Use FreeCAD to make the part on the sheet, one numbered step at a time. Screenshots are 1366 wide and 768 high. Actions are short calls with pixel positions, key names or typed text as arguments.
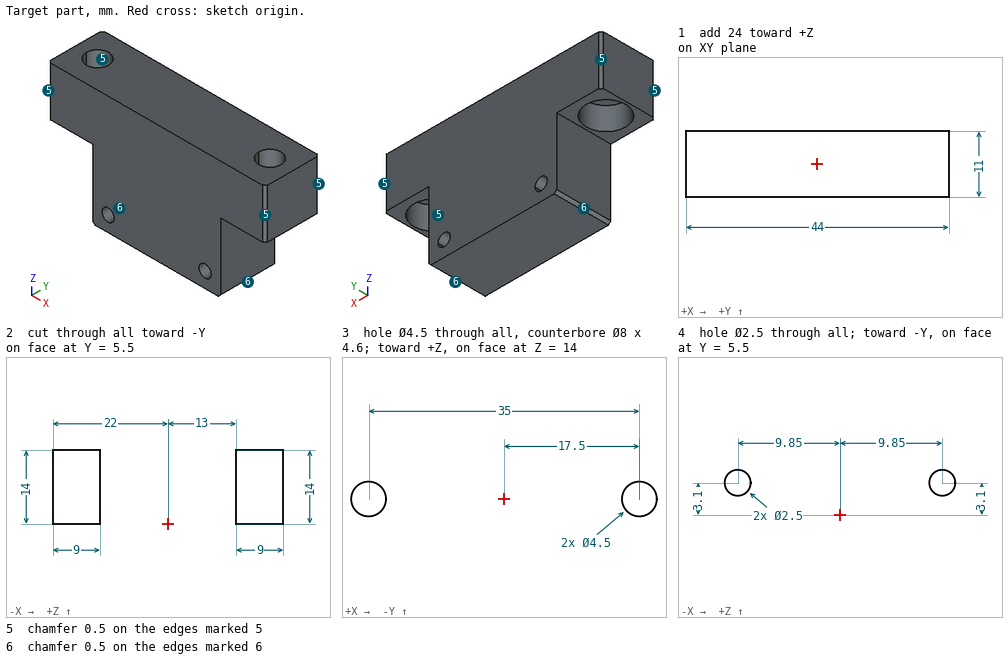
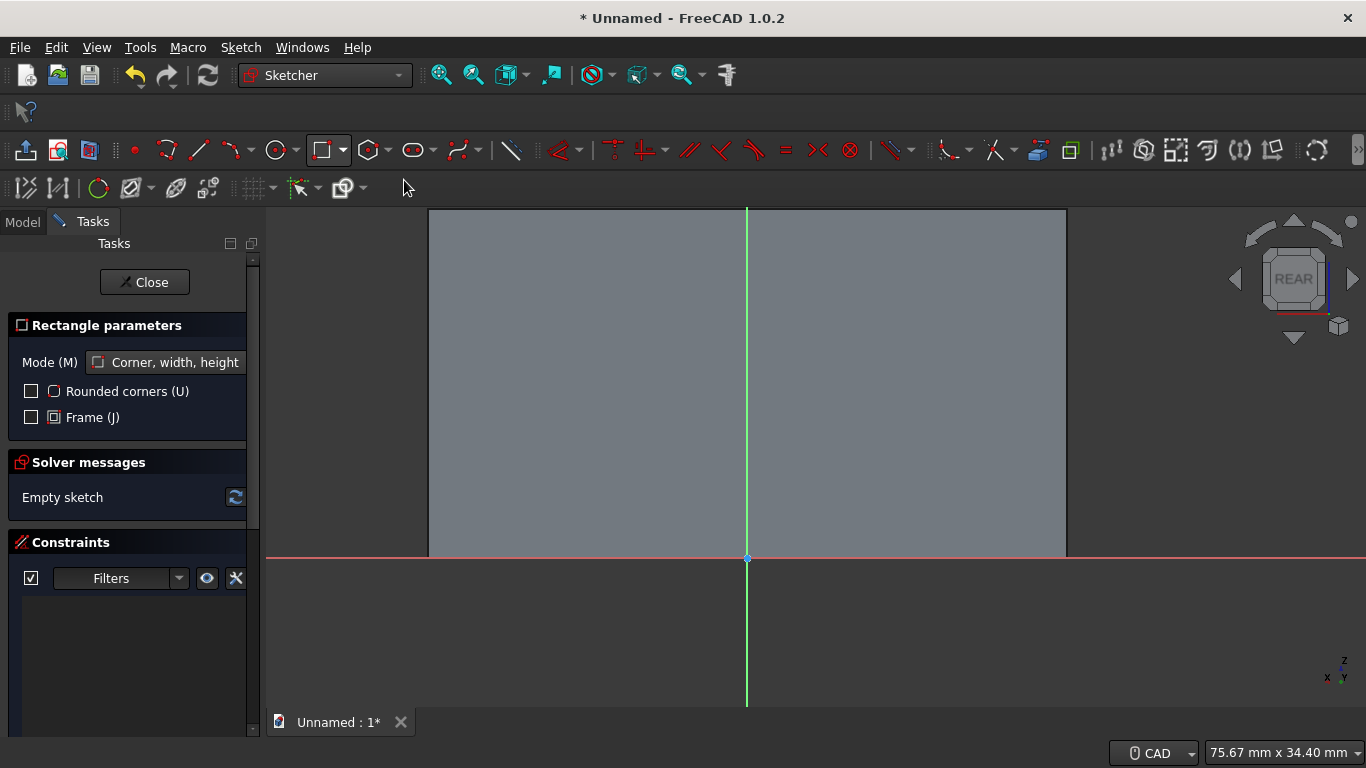
click(936, 355)
click(1067, 558)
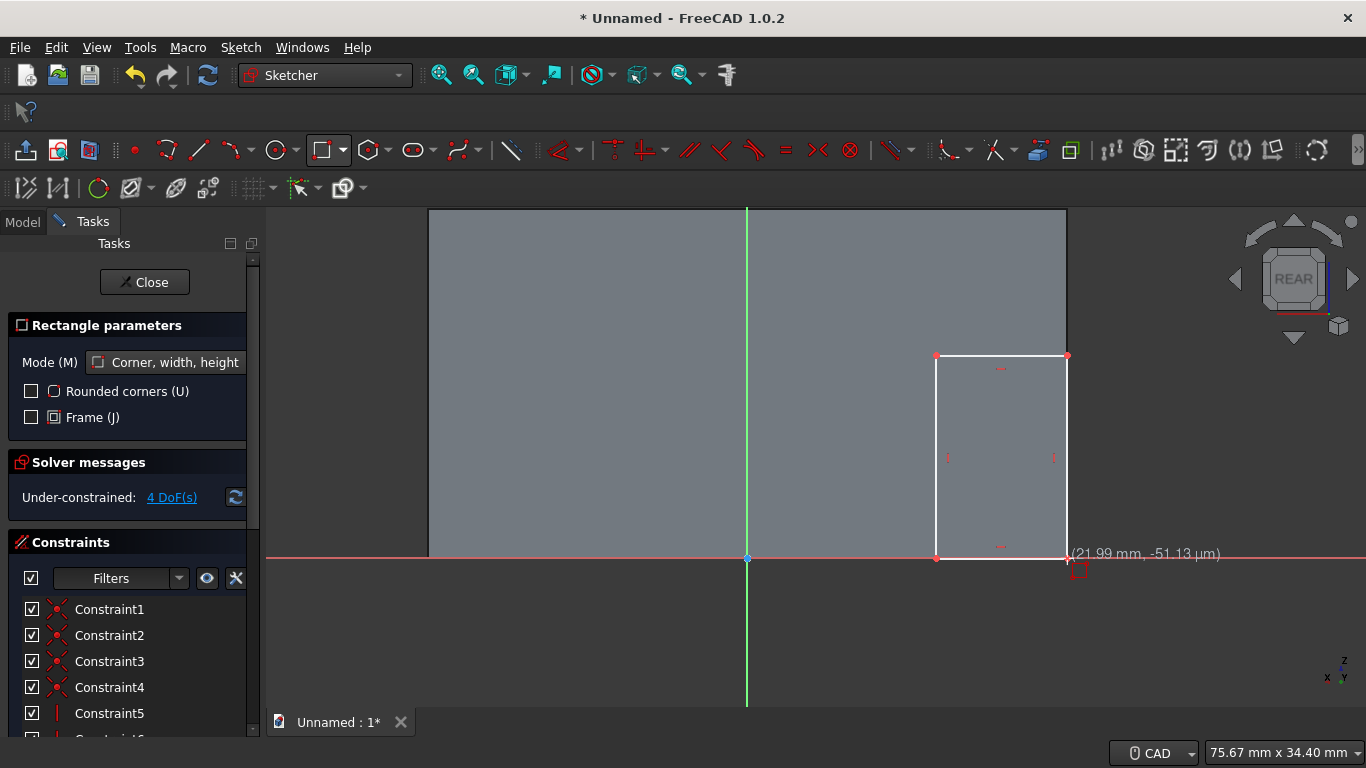
click(428, 355)
click(558, 558)
key(Escape)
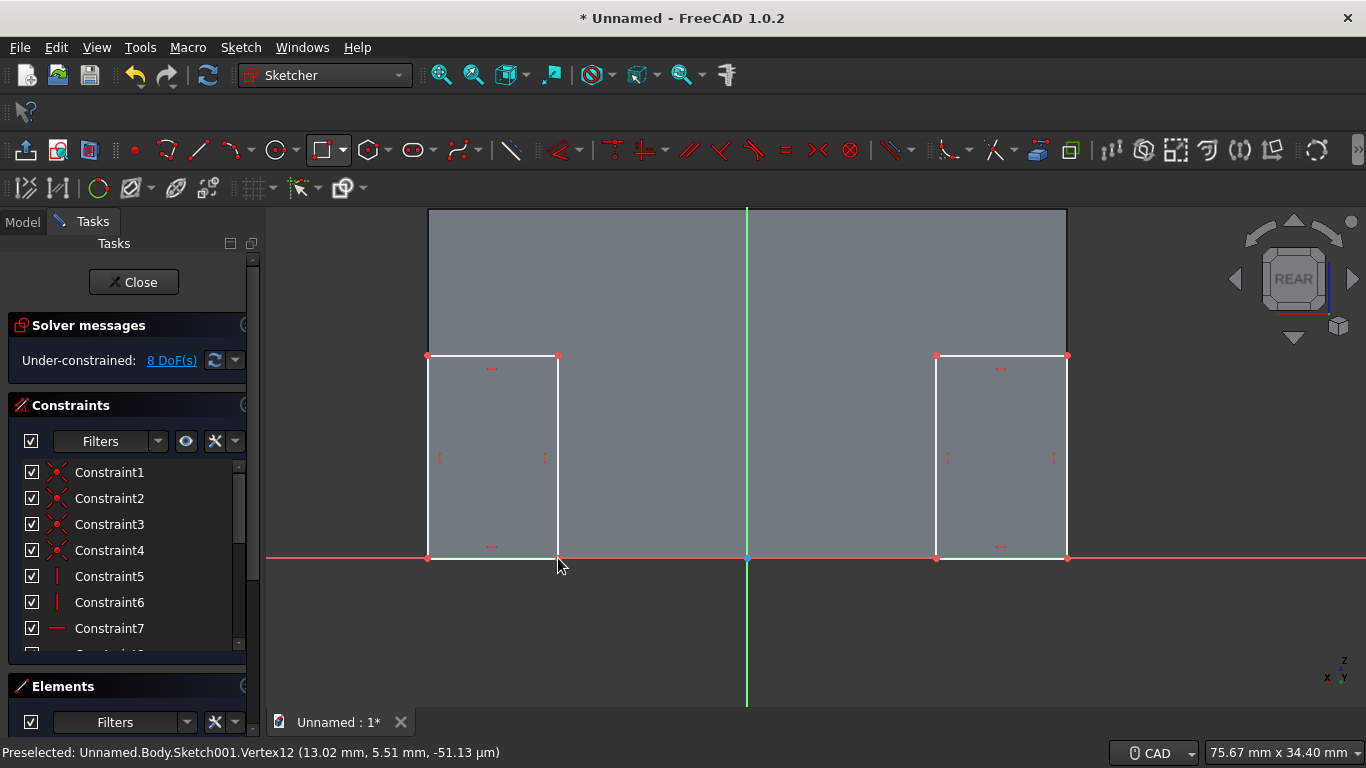
click(936, 559)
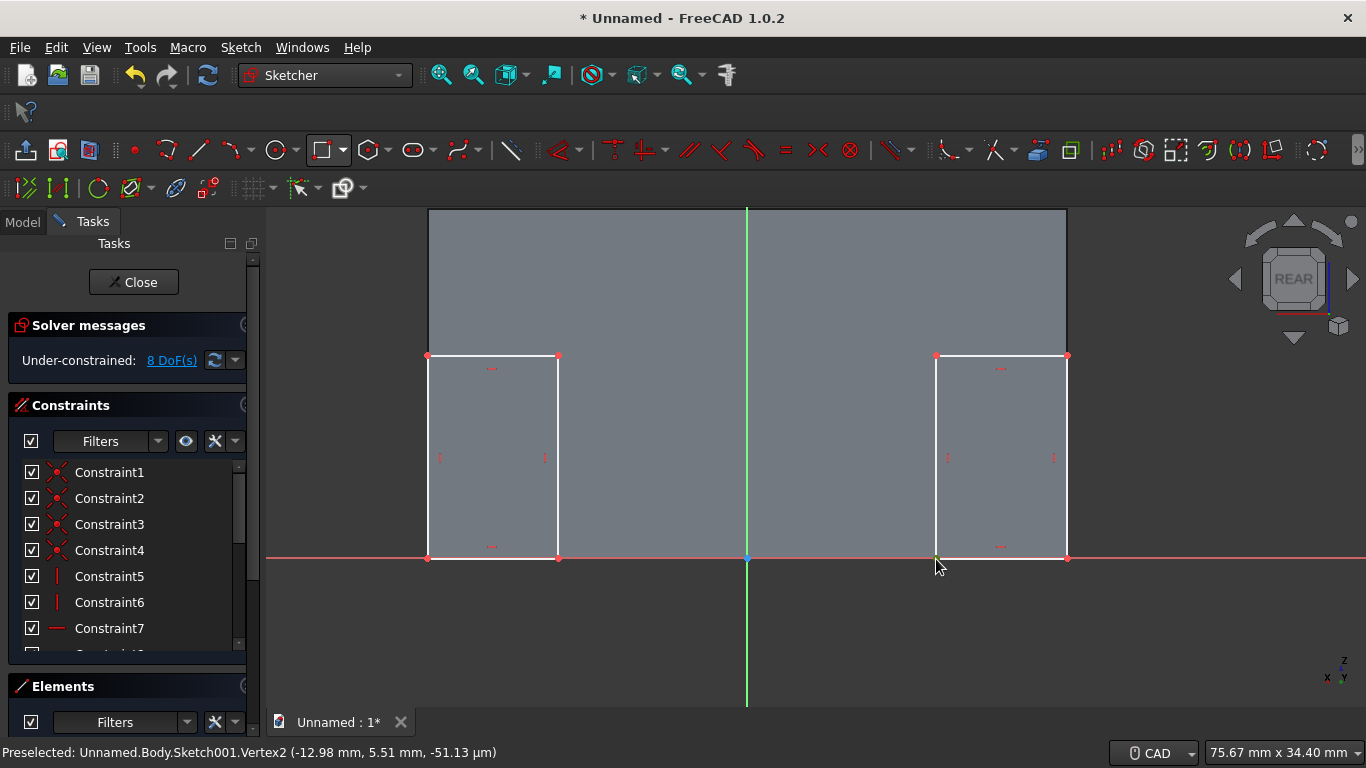
click(359, 558)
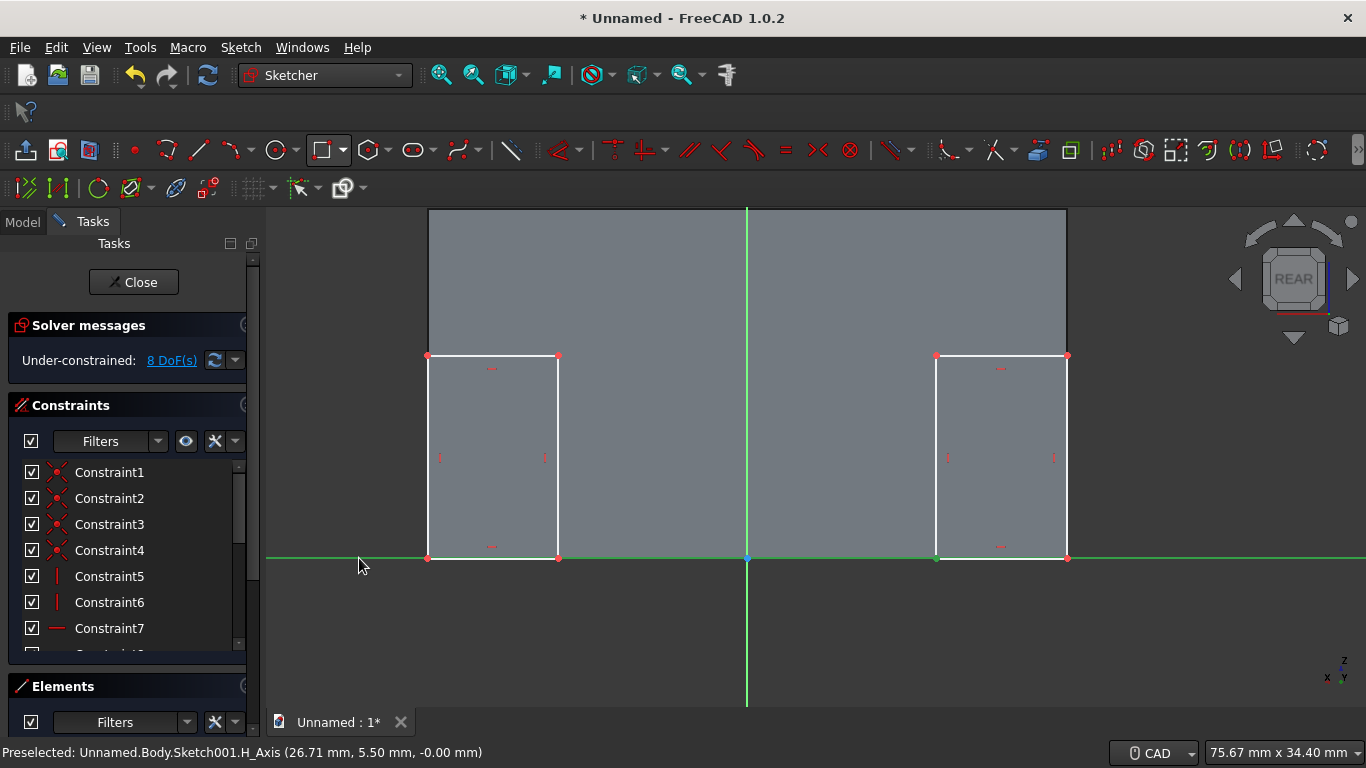
click(614, 150)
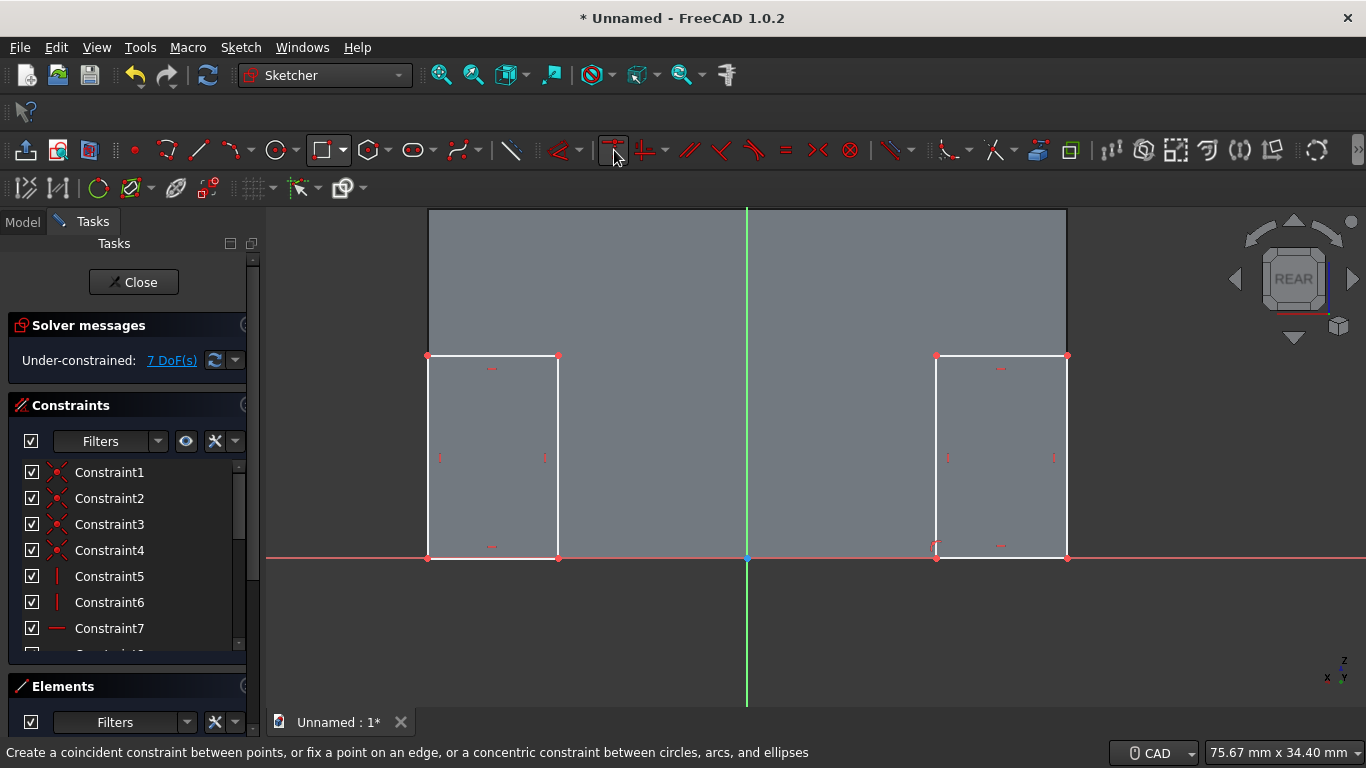
click(428, 559)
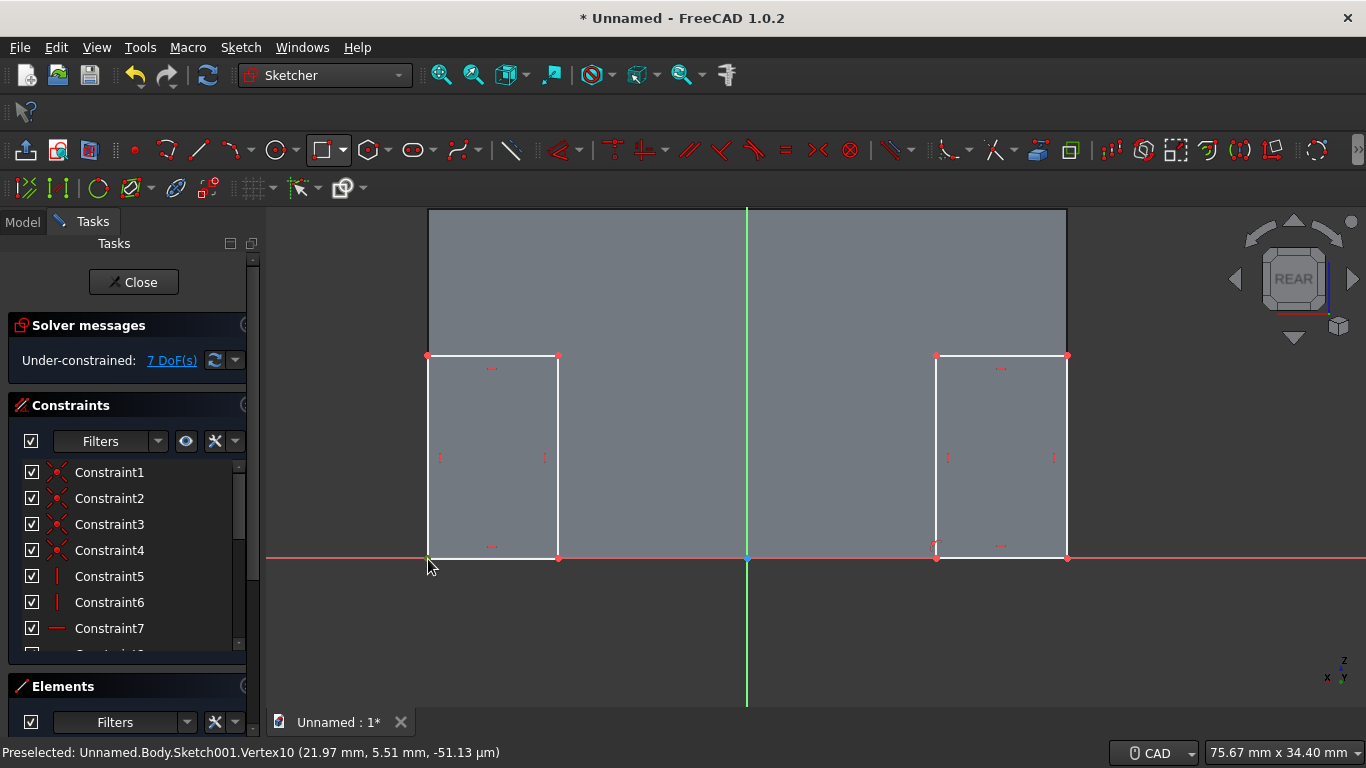
click(359, 558)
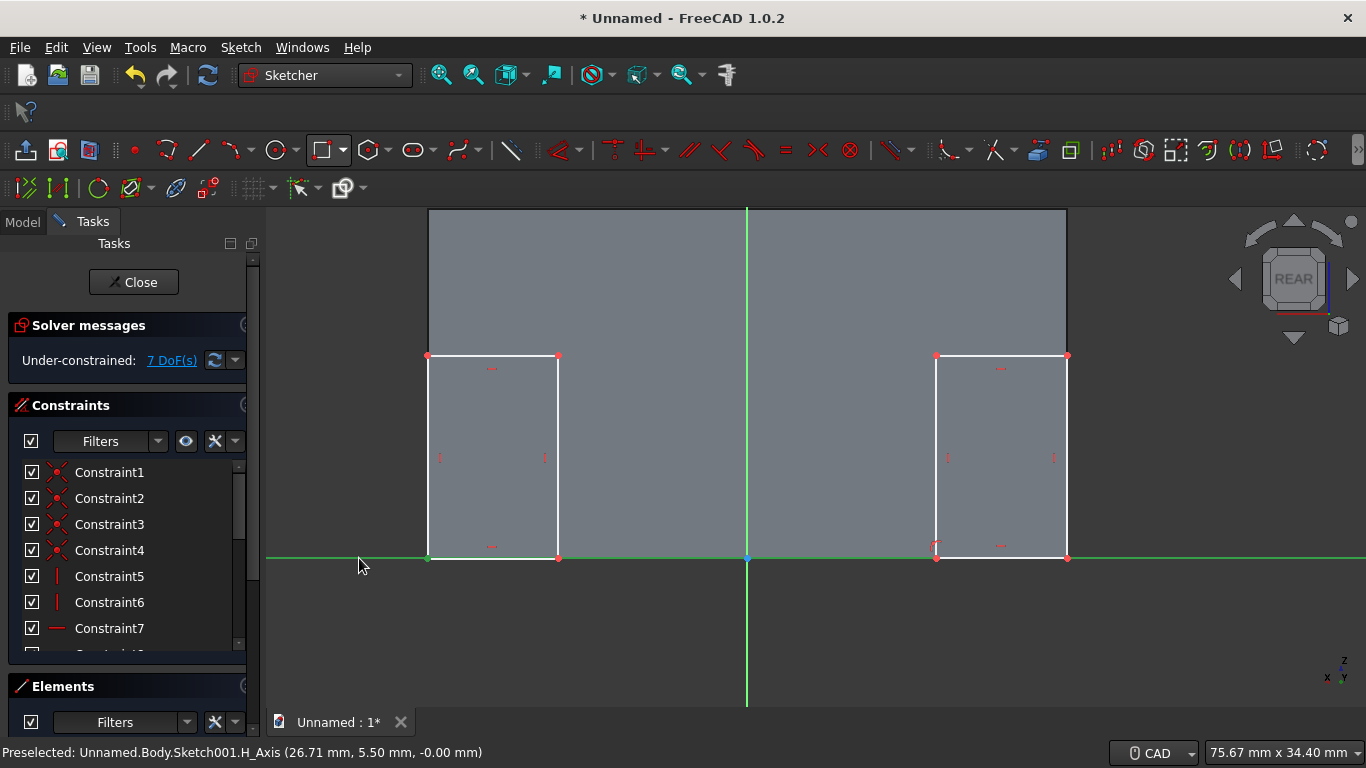
click(614, 150)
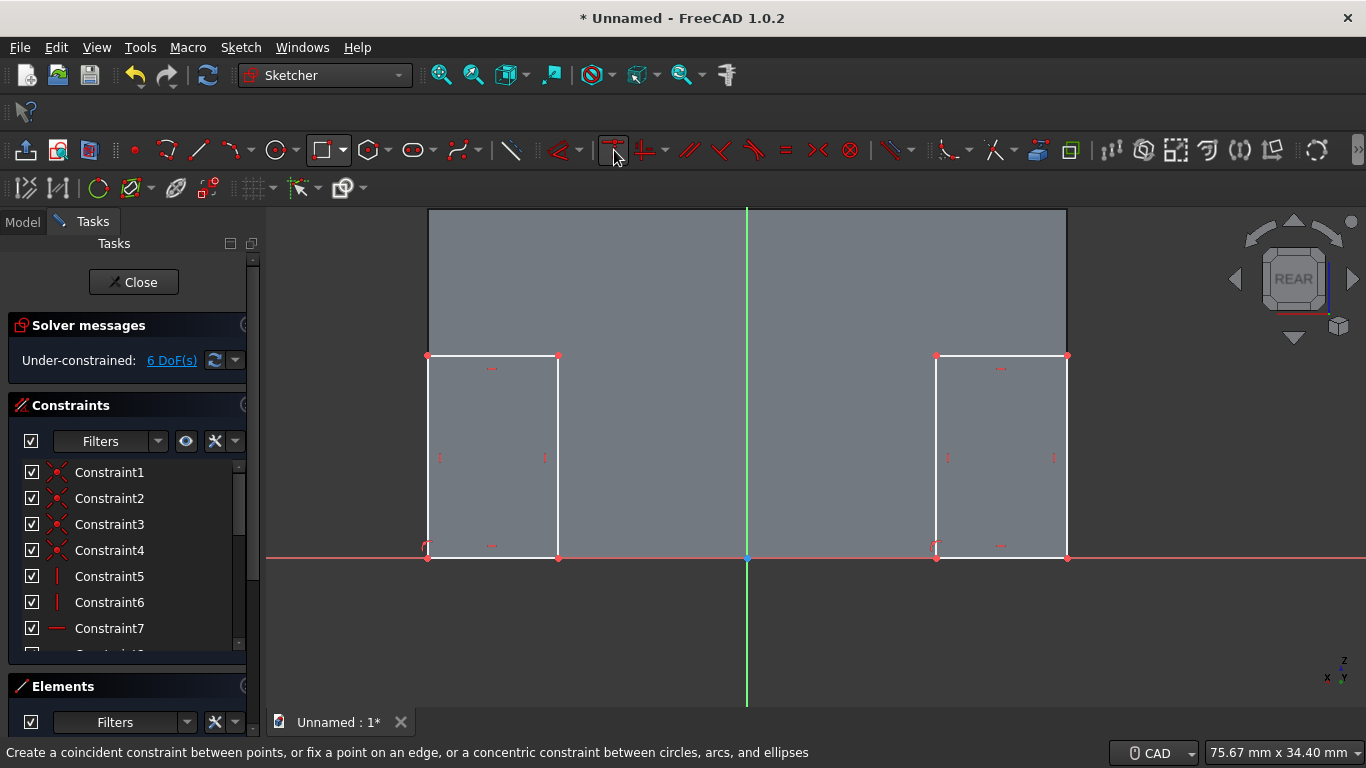
click(558, 150)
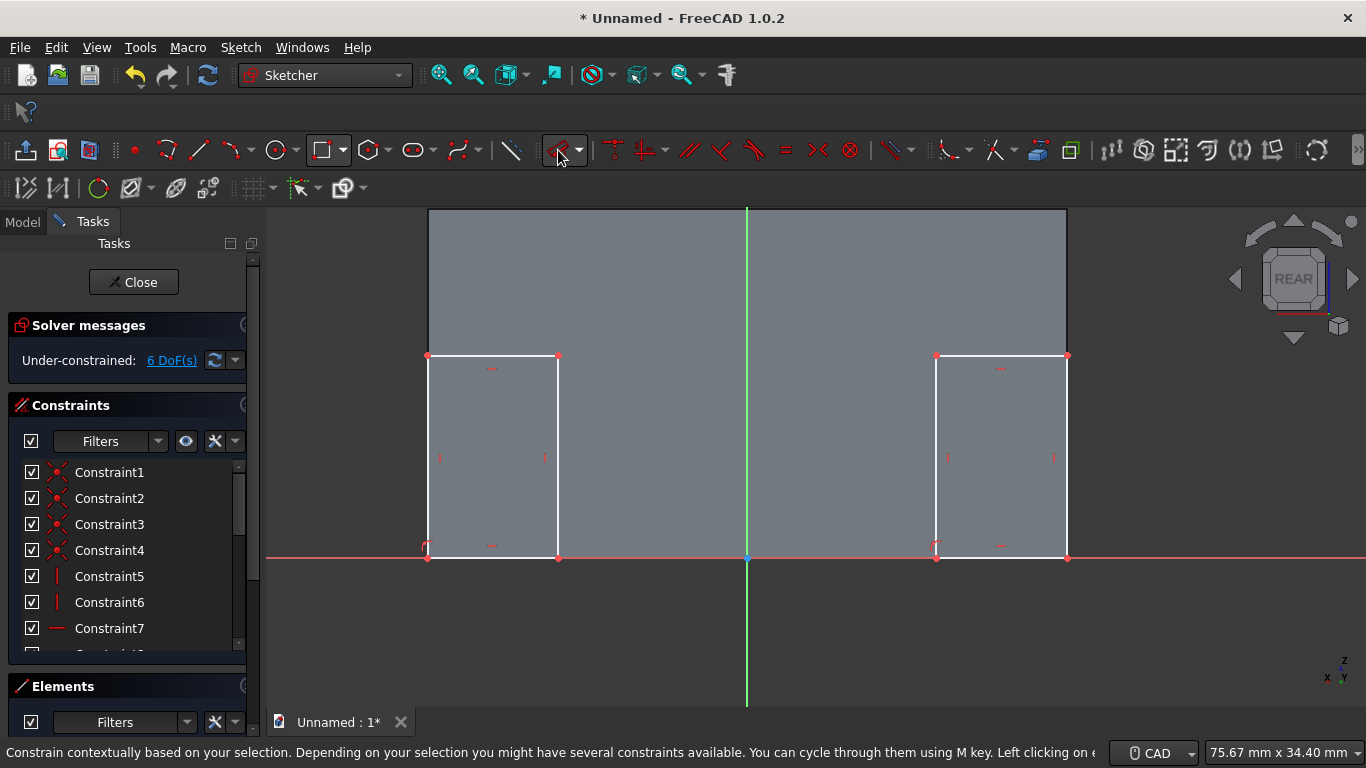
click(975, 558)
click(1002, 592)